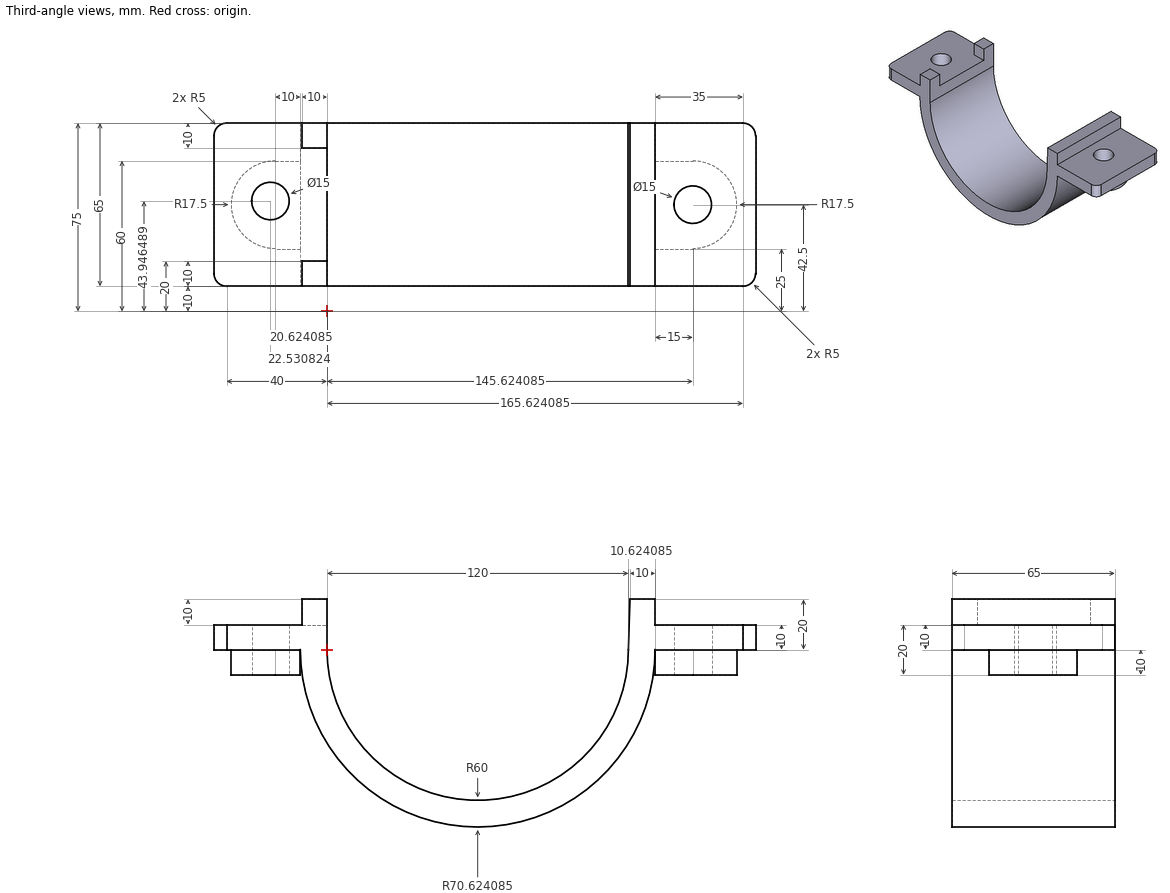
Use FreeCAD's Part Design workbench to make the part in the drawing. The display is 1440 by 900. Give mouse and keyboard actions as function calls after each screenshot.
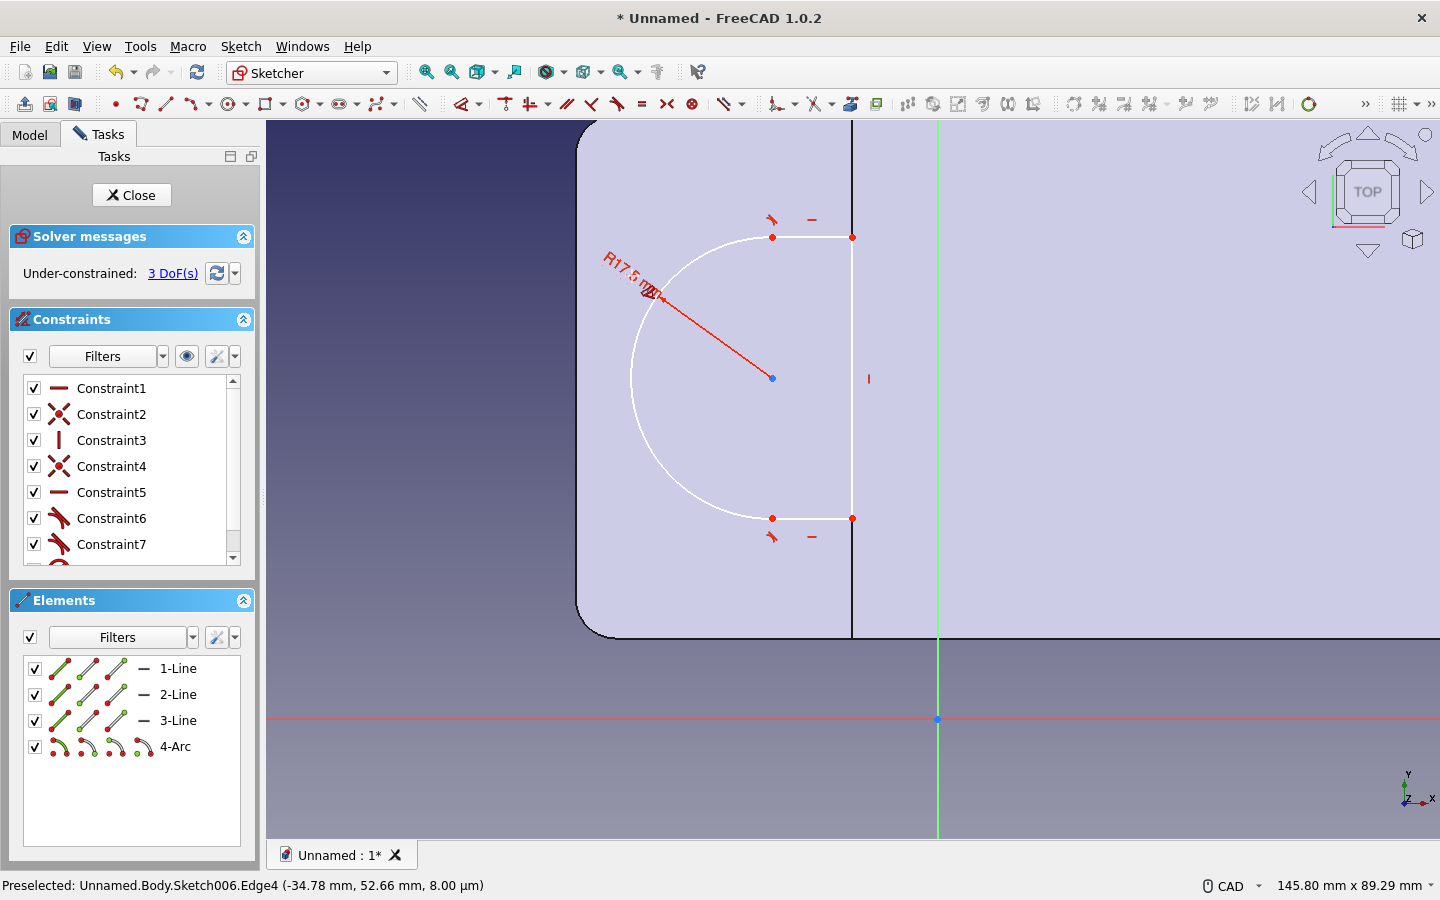
click(796, 237)
click(812, 203)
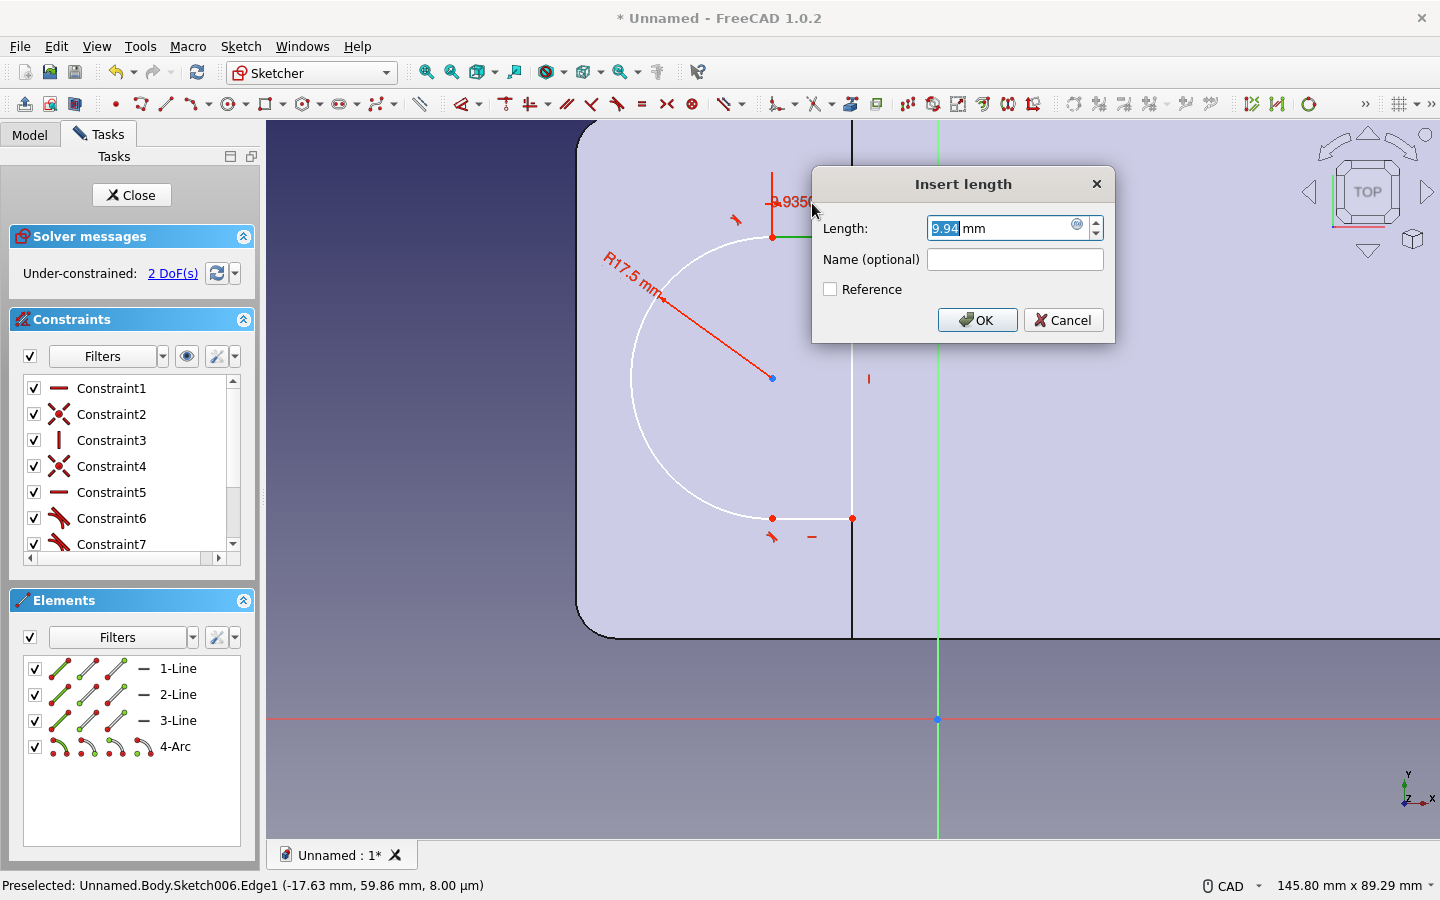
text(10)
key(Return)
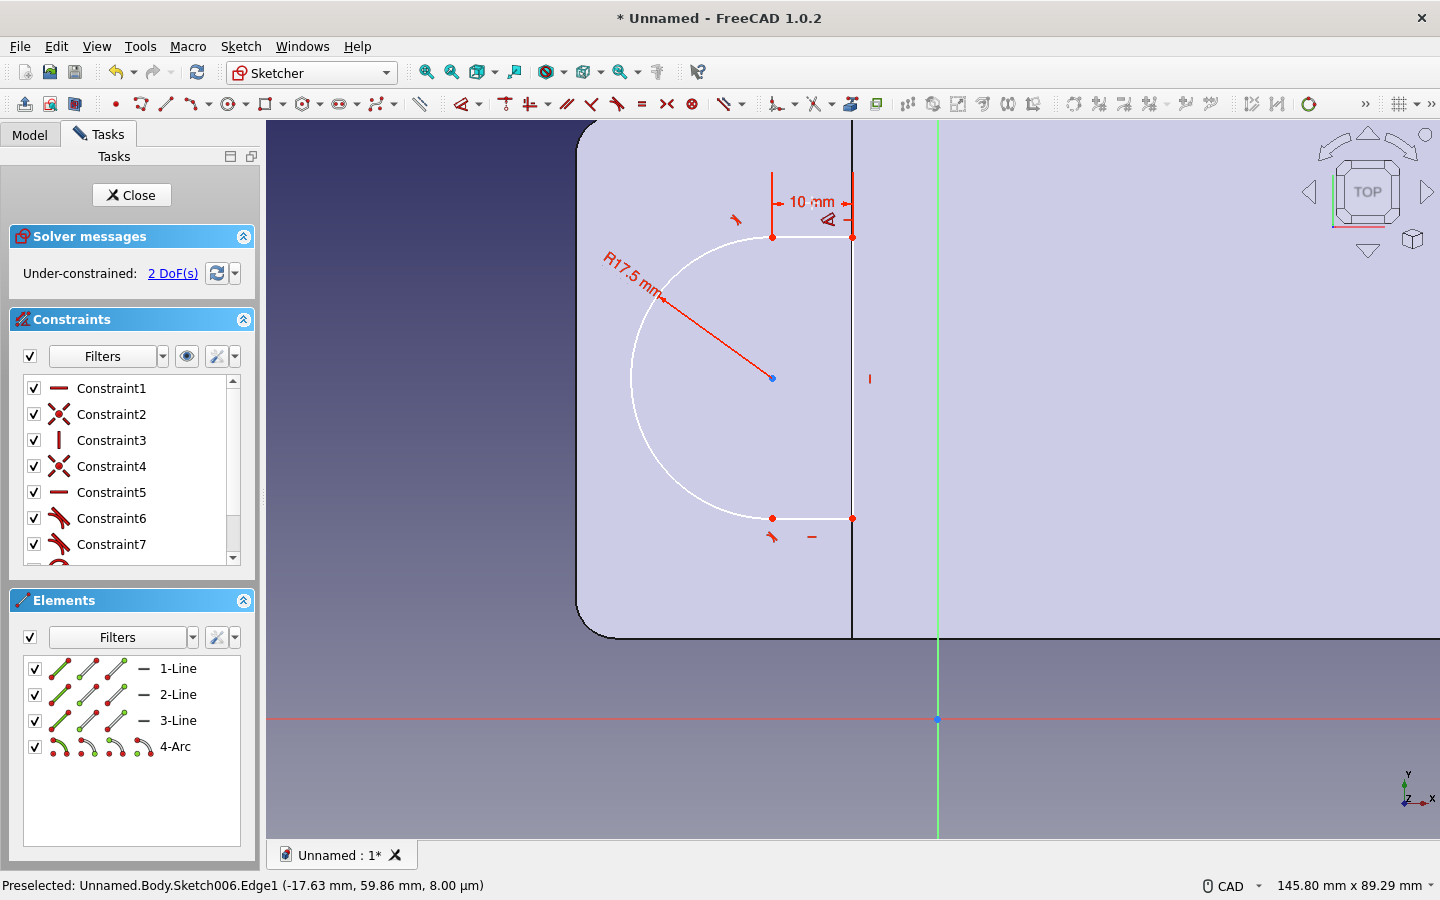
click(772, 237)
click(972, 478)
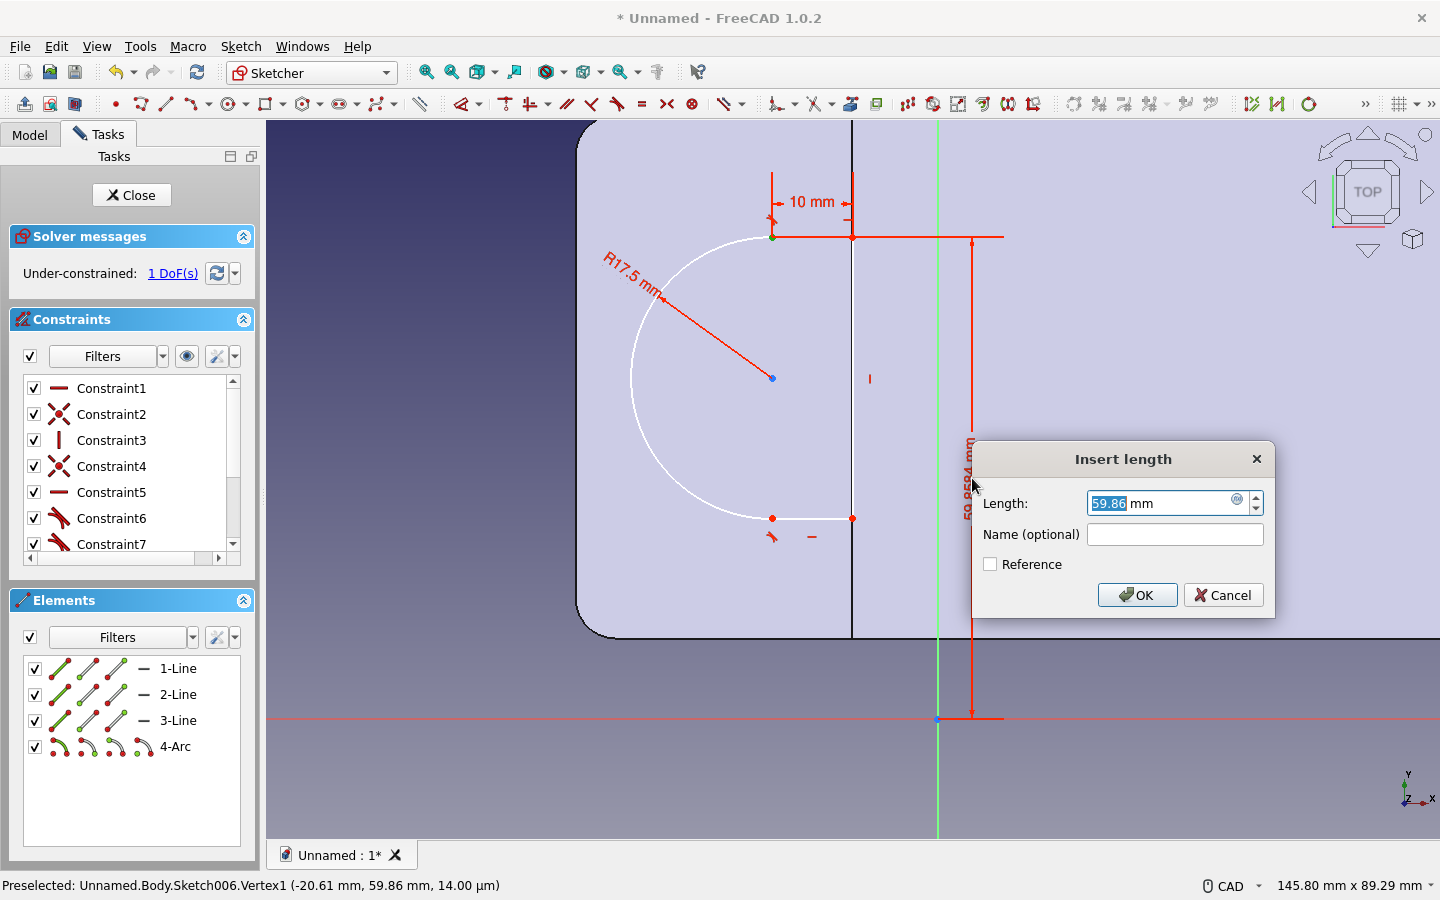
text(60)
key(Return)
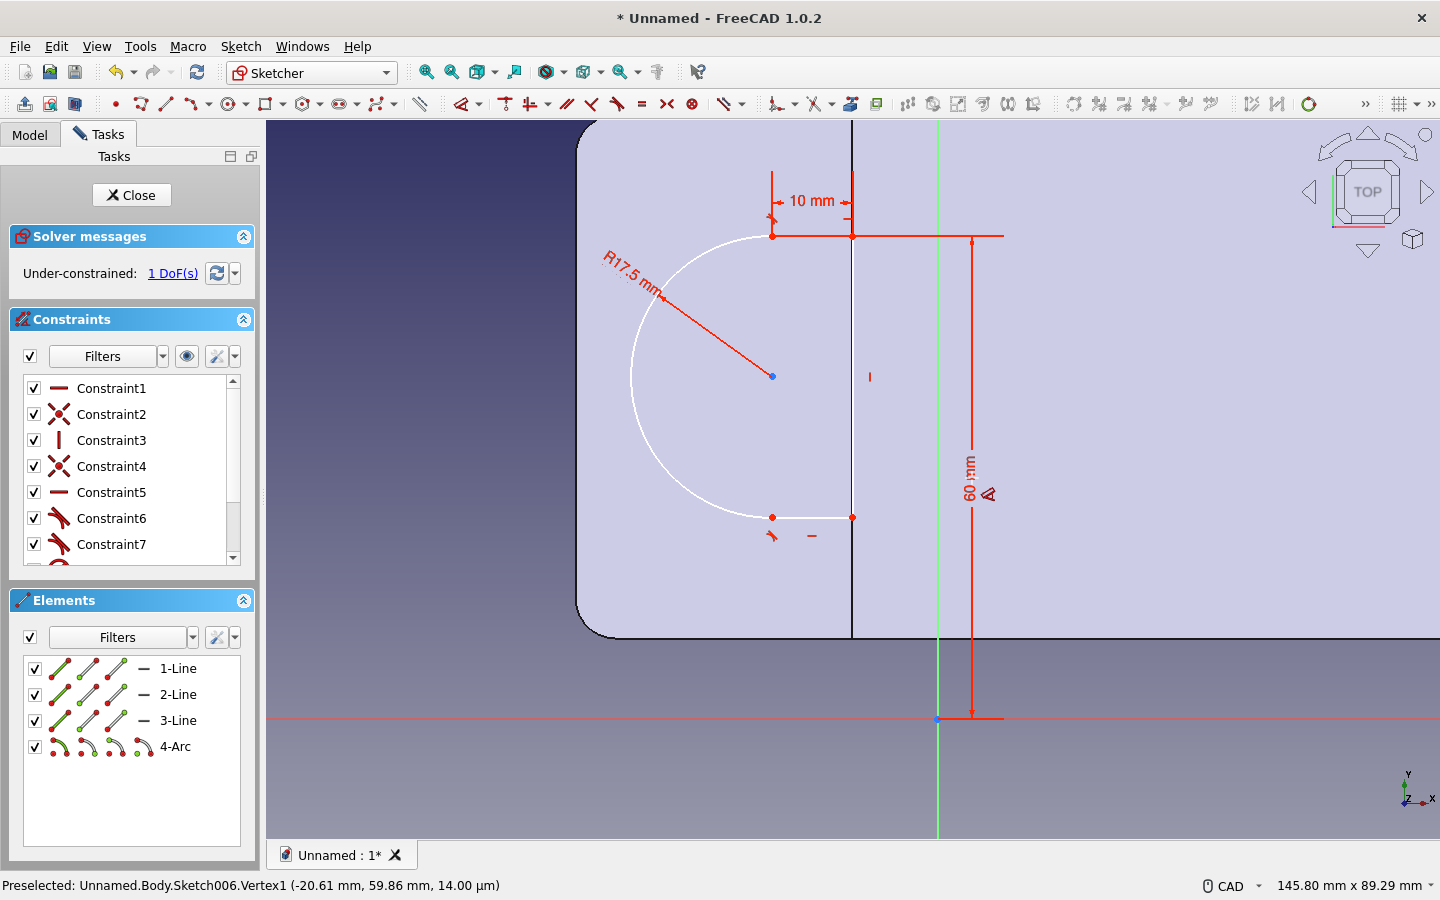
click(772, 236)
click(855, 753)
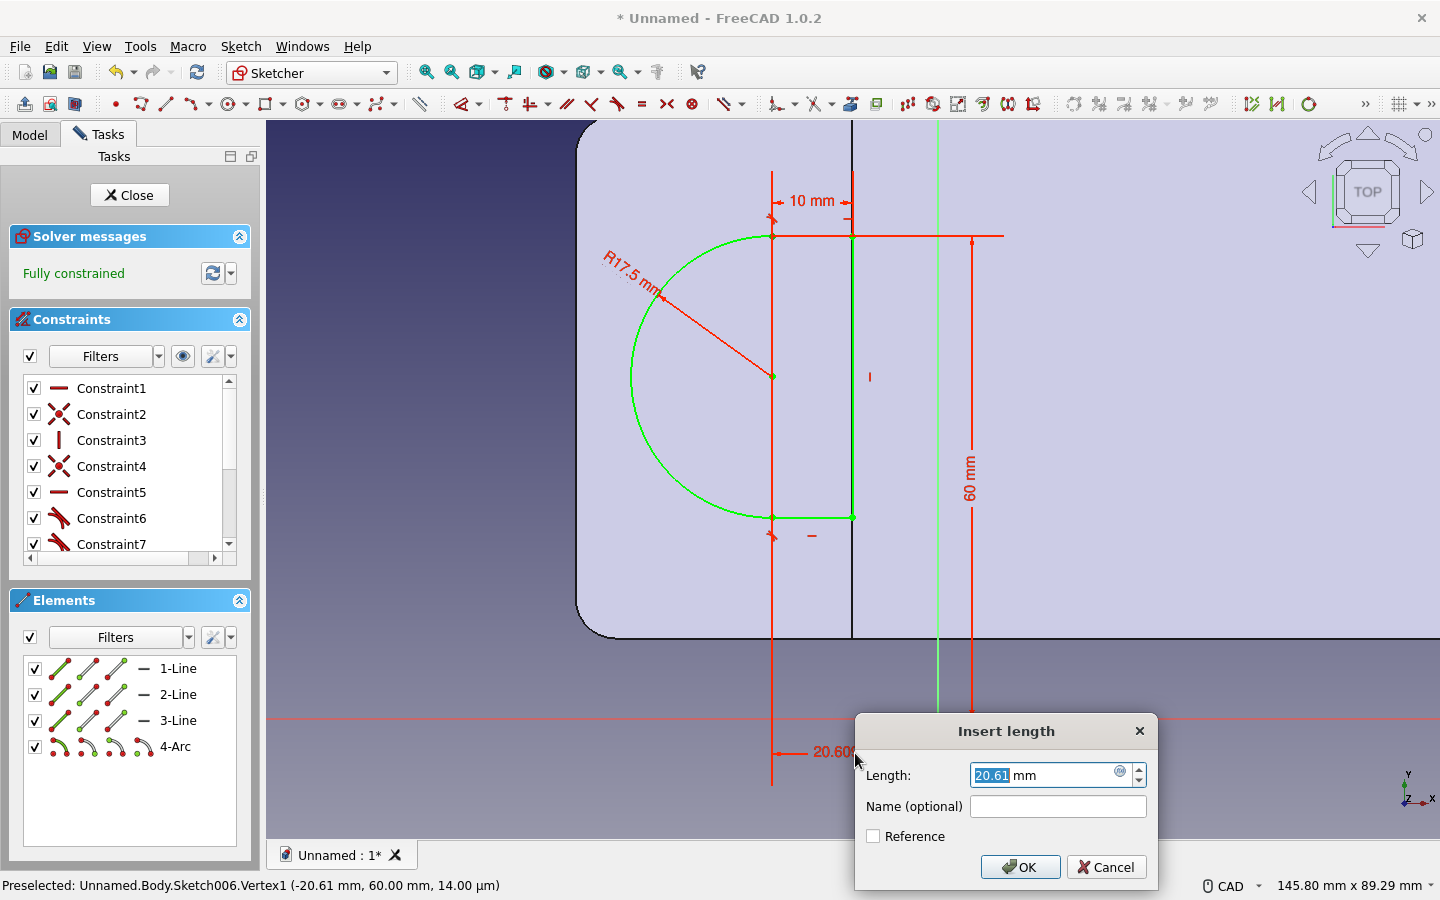
text(20.624085)
key(Return)
key(Escape)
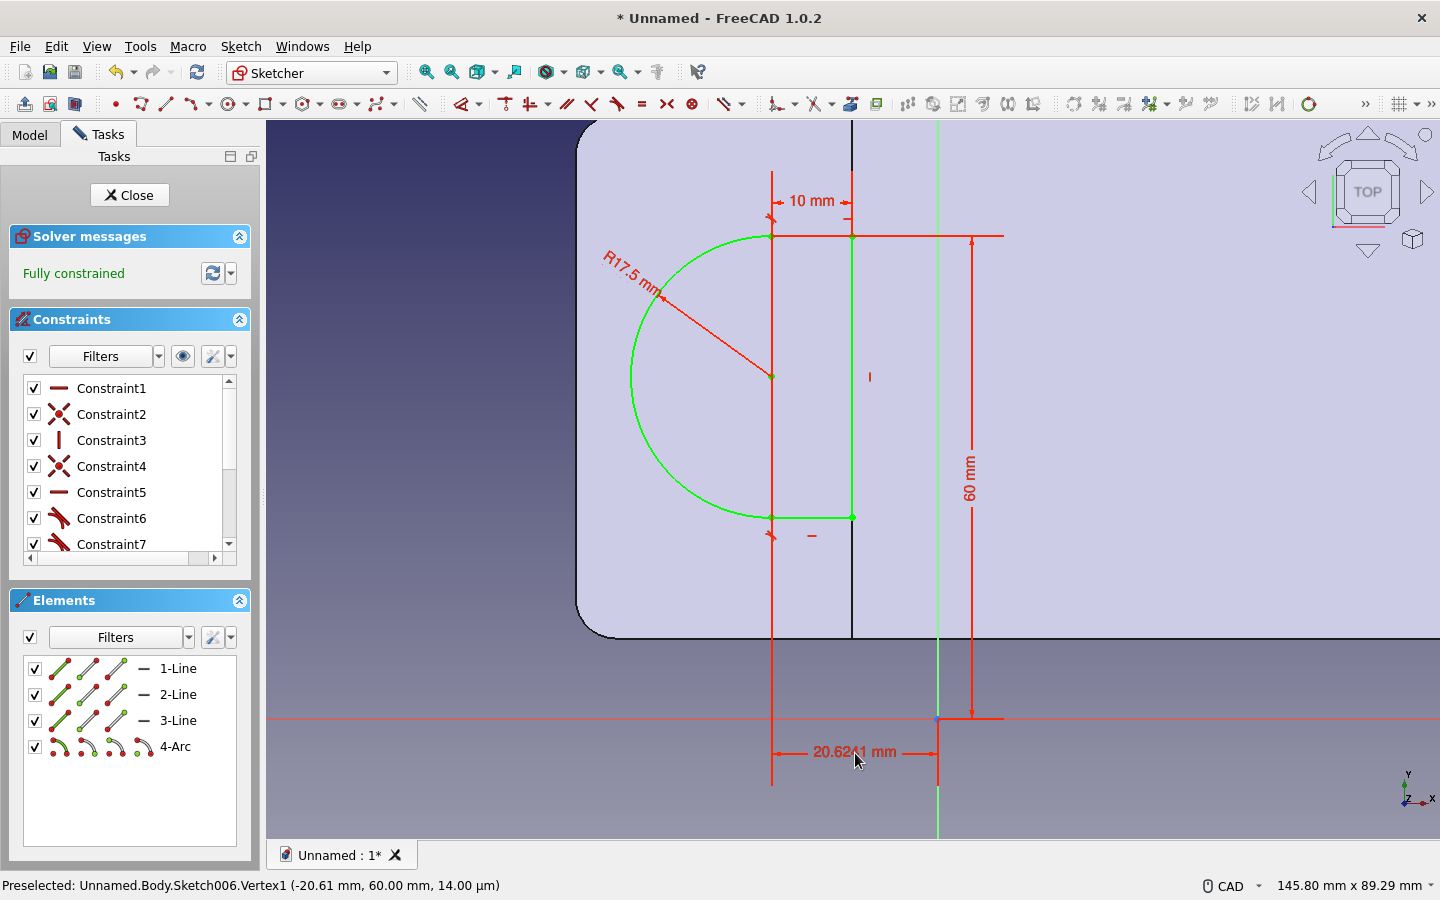
click(130, 195)